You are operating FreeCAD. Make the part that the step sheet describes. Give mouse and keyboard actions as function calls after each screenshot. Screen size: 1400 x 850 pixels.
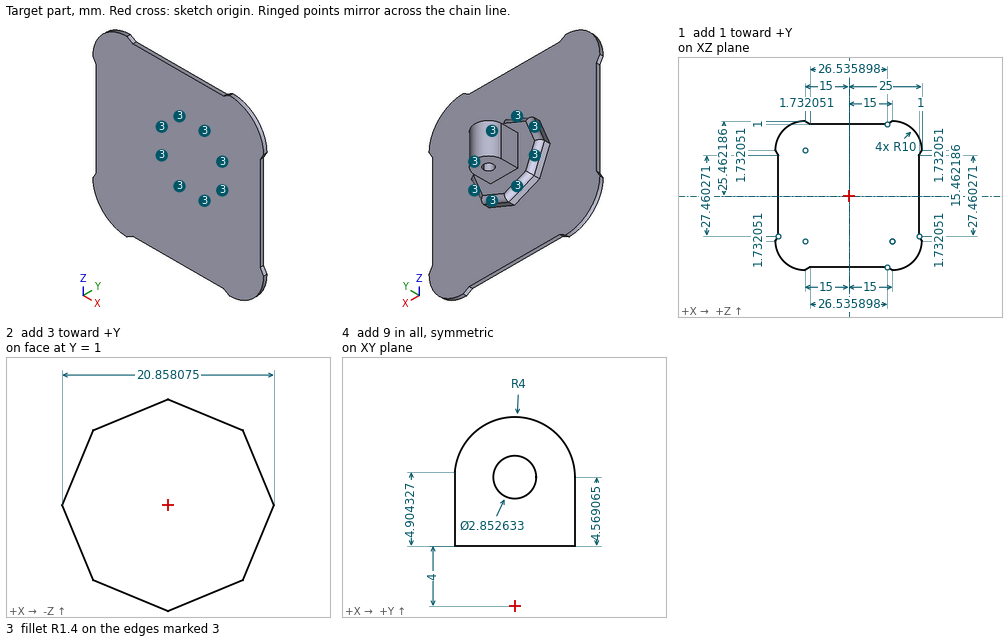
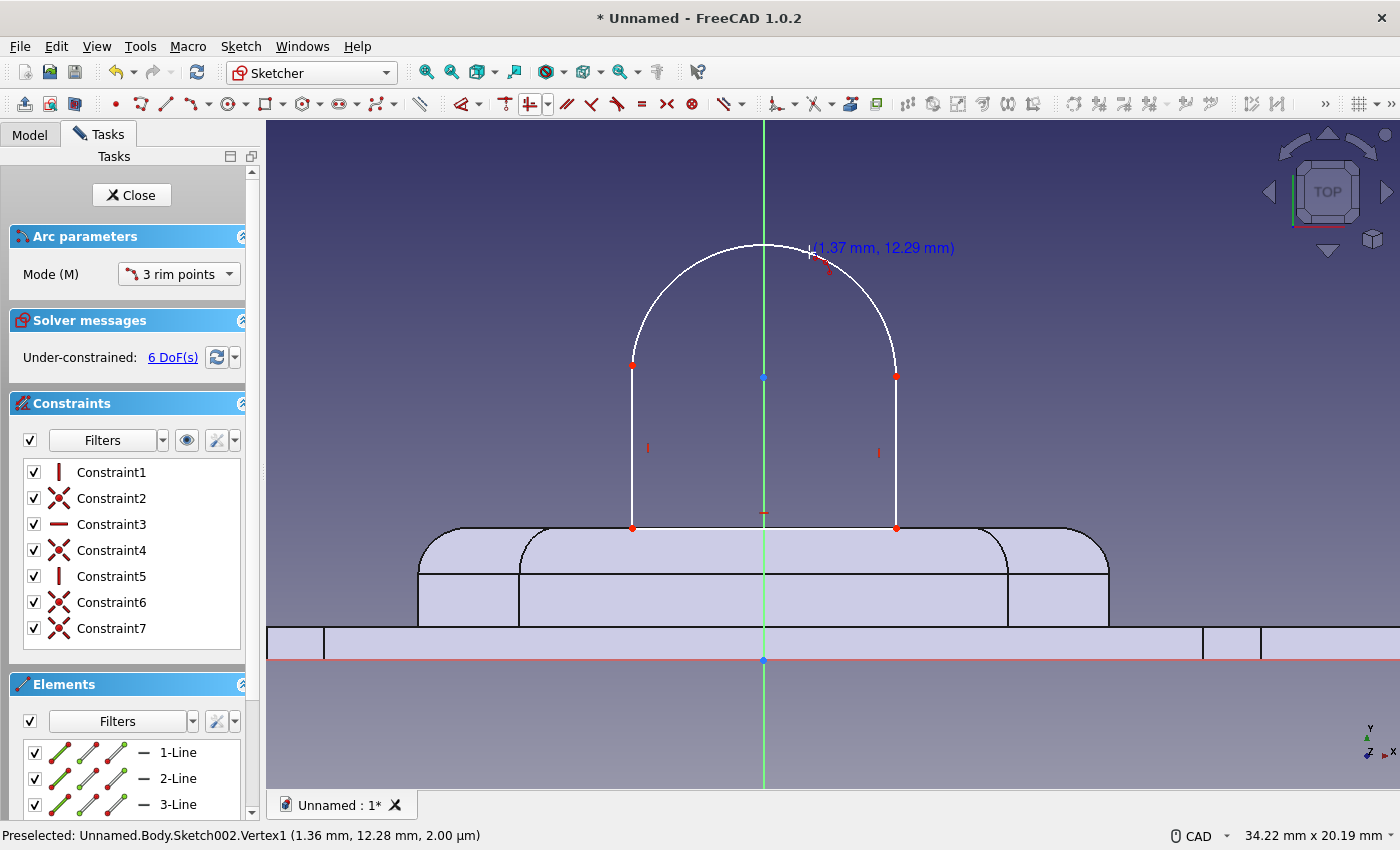
click(228, 104)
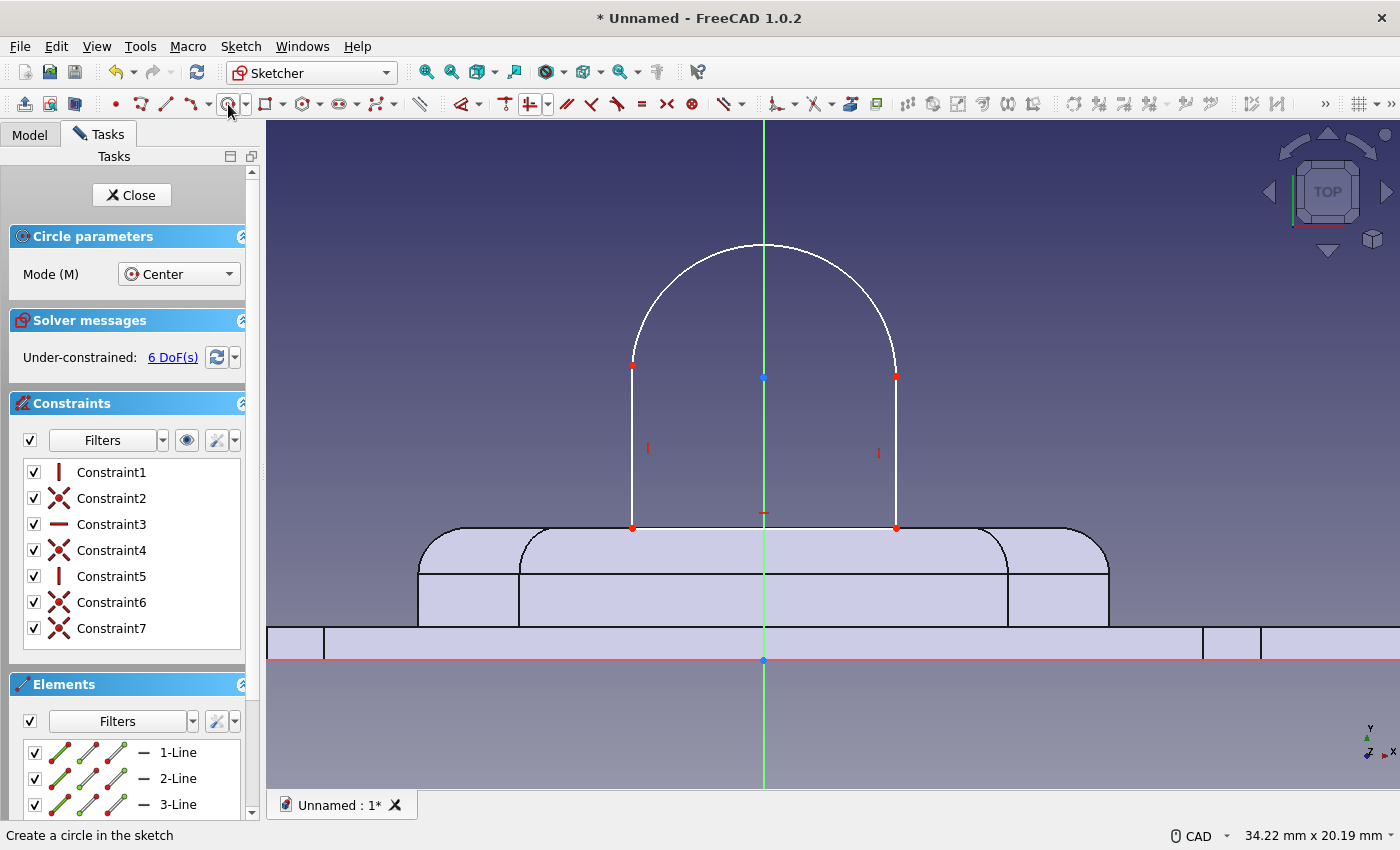
click(764, 376)
click(797, 343)
key(Escape)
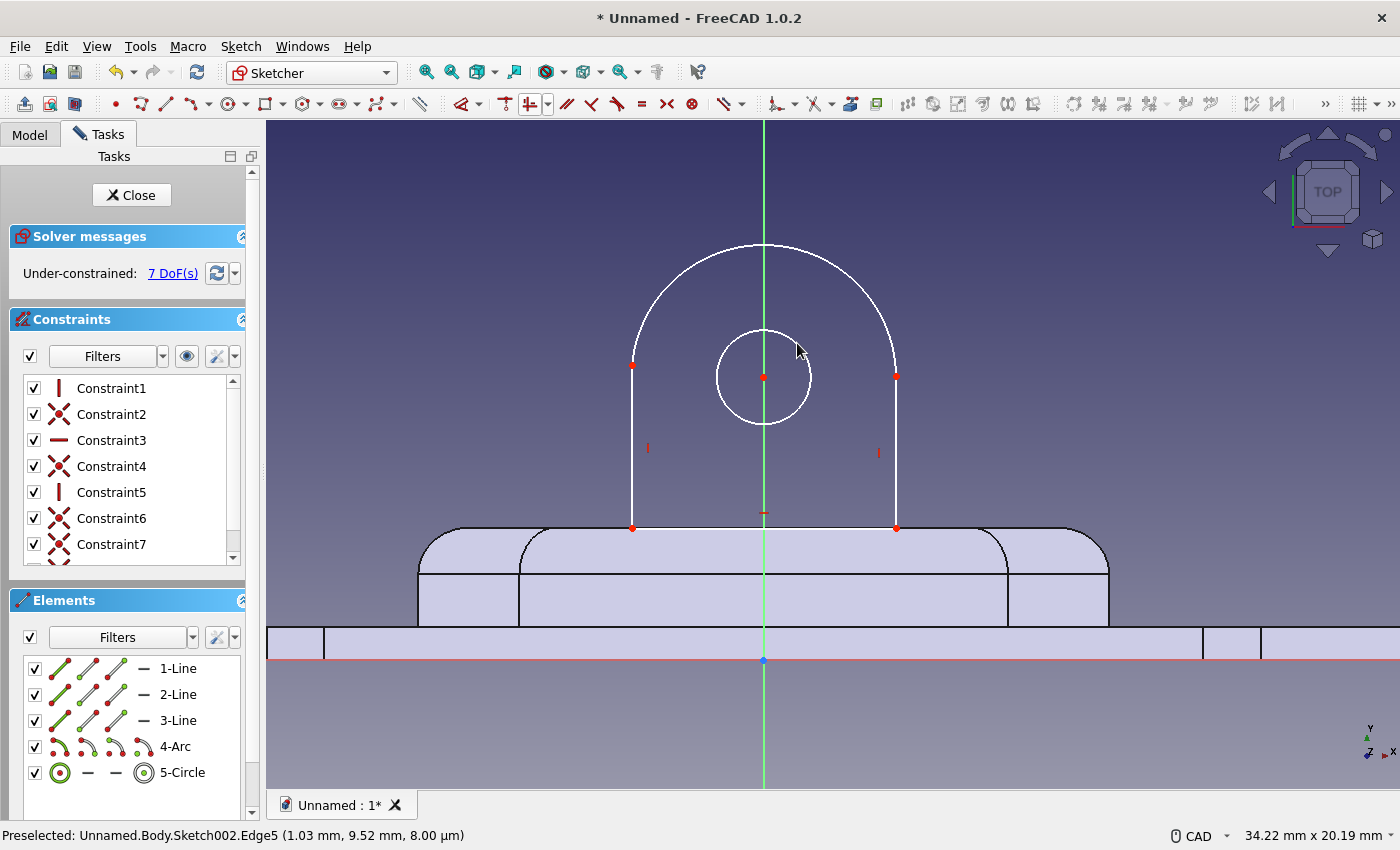
click(896, 483)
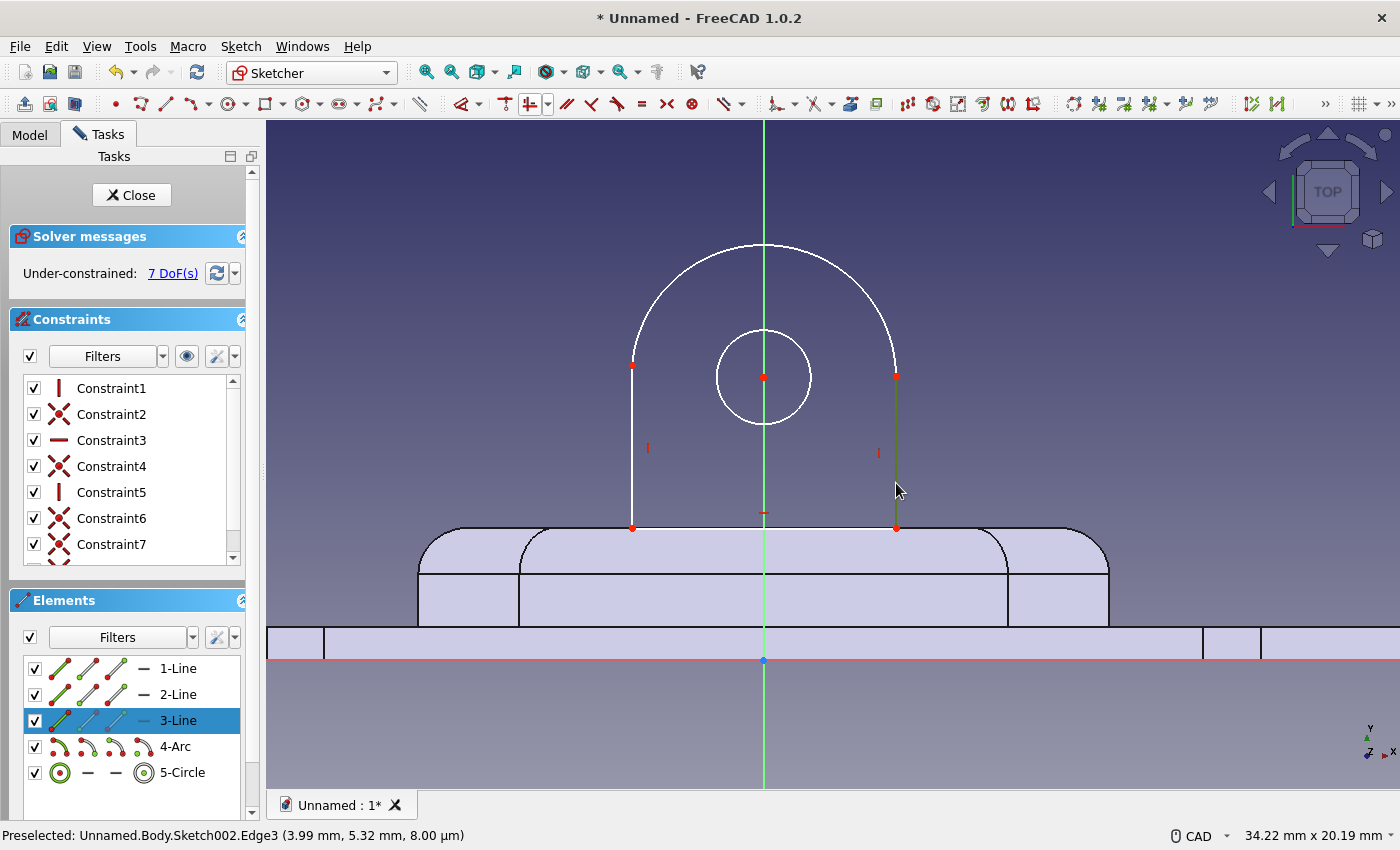
click(844, 272)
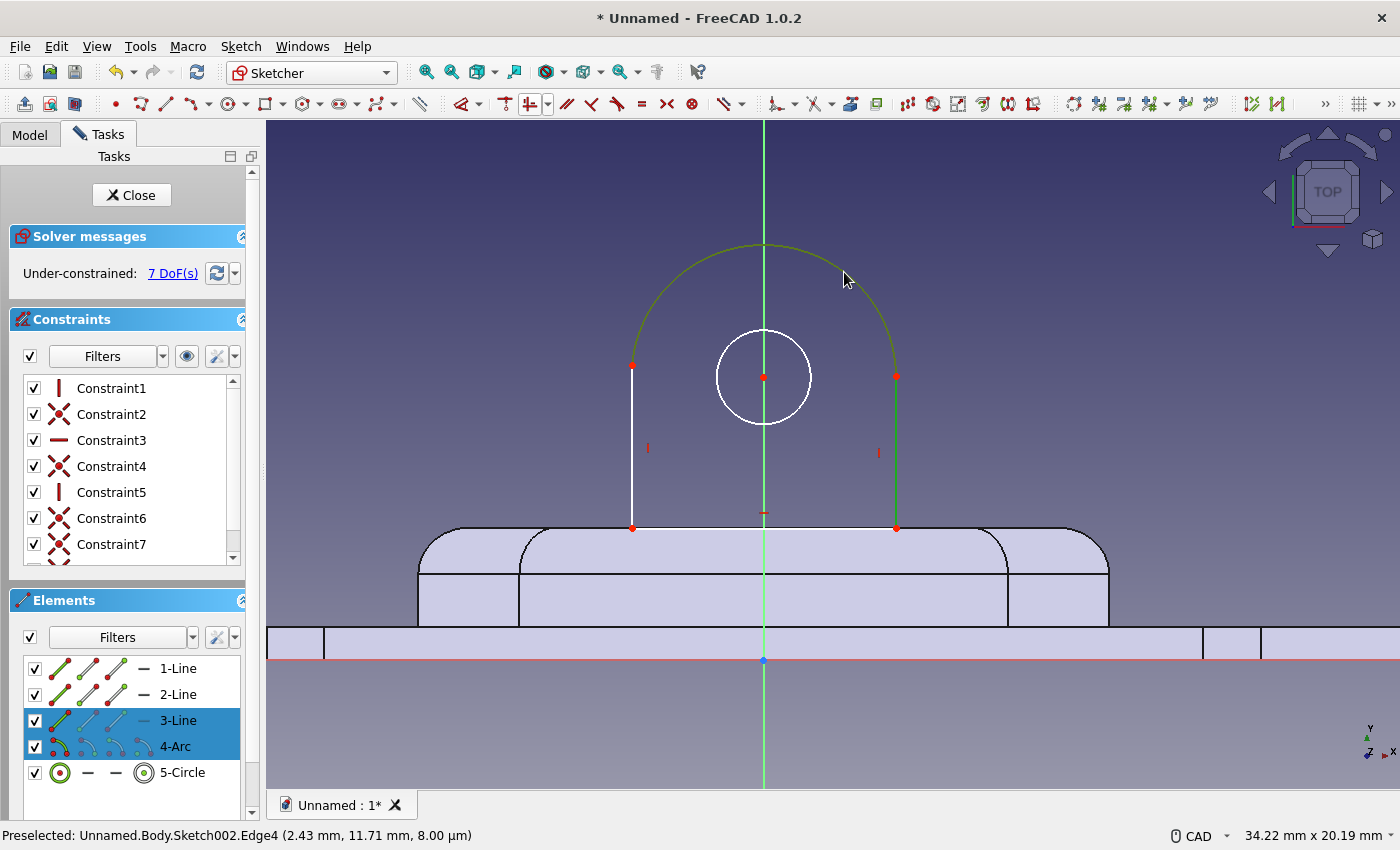
click(617, 104)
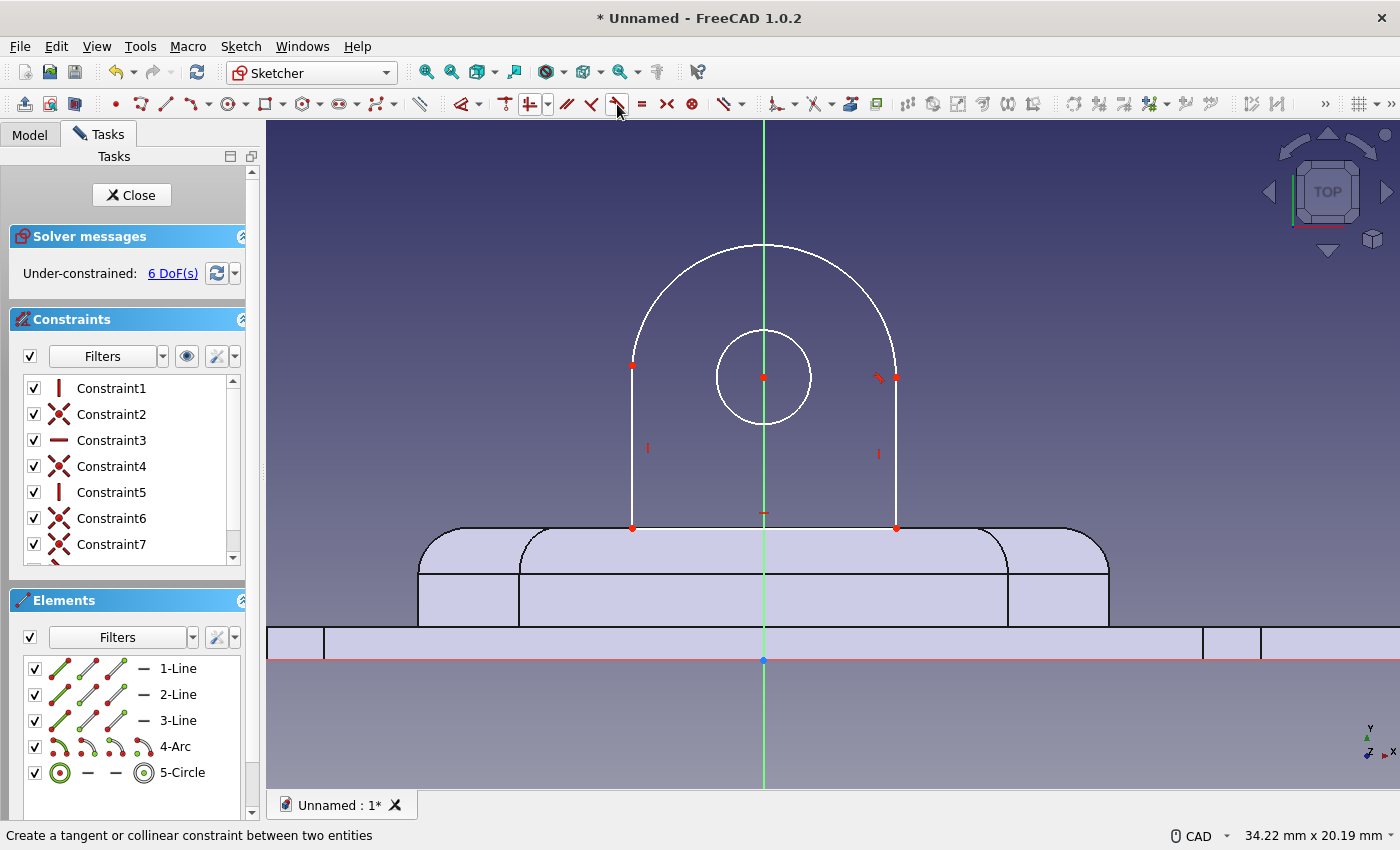
click(764, 377)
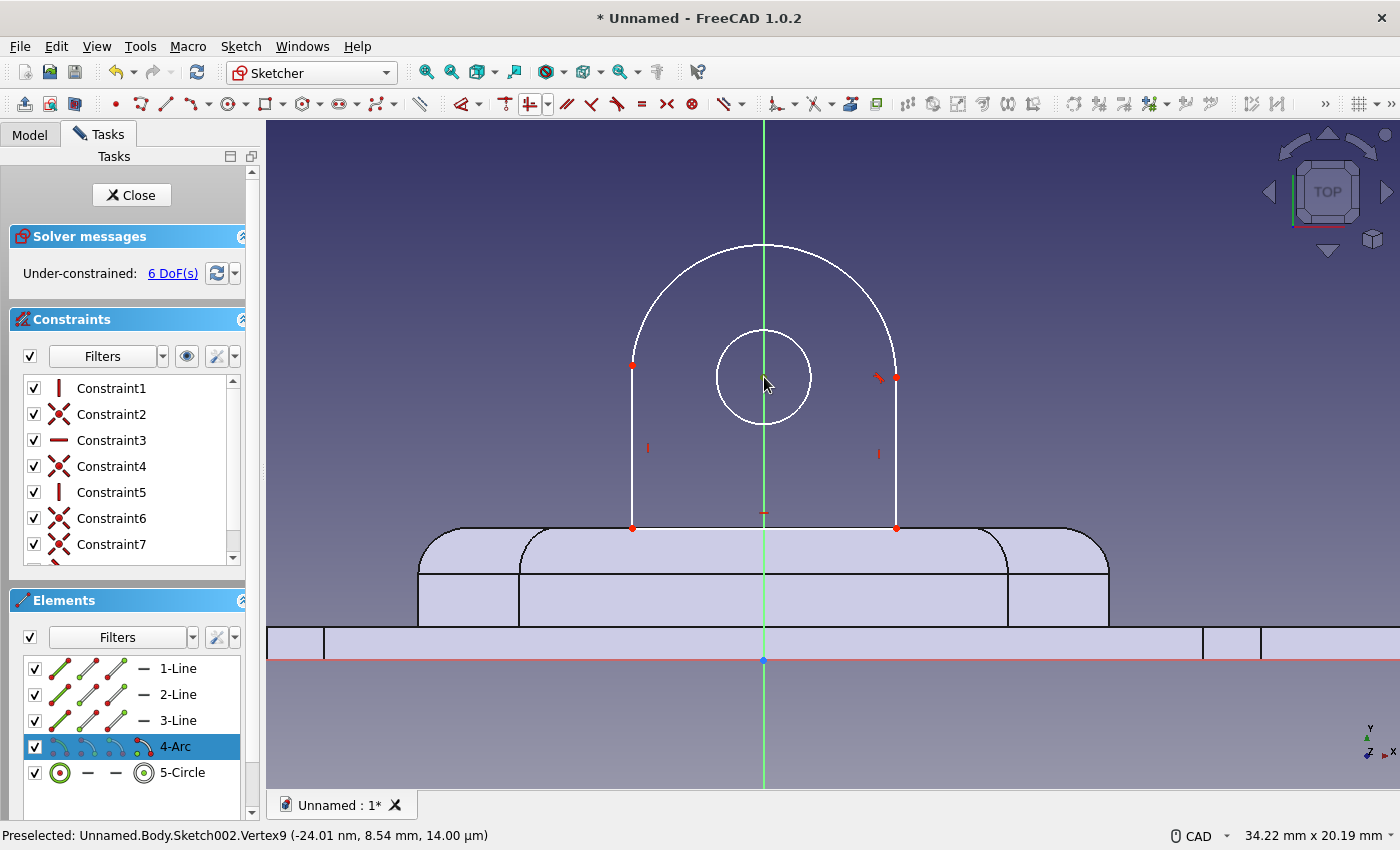
click(764, 717)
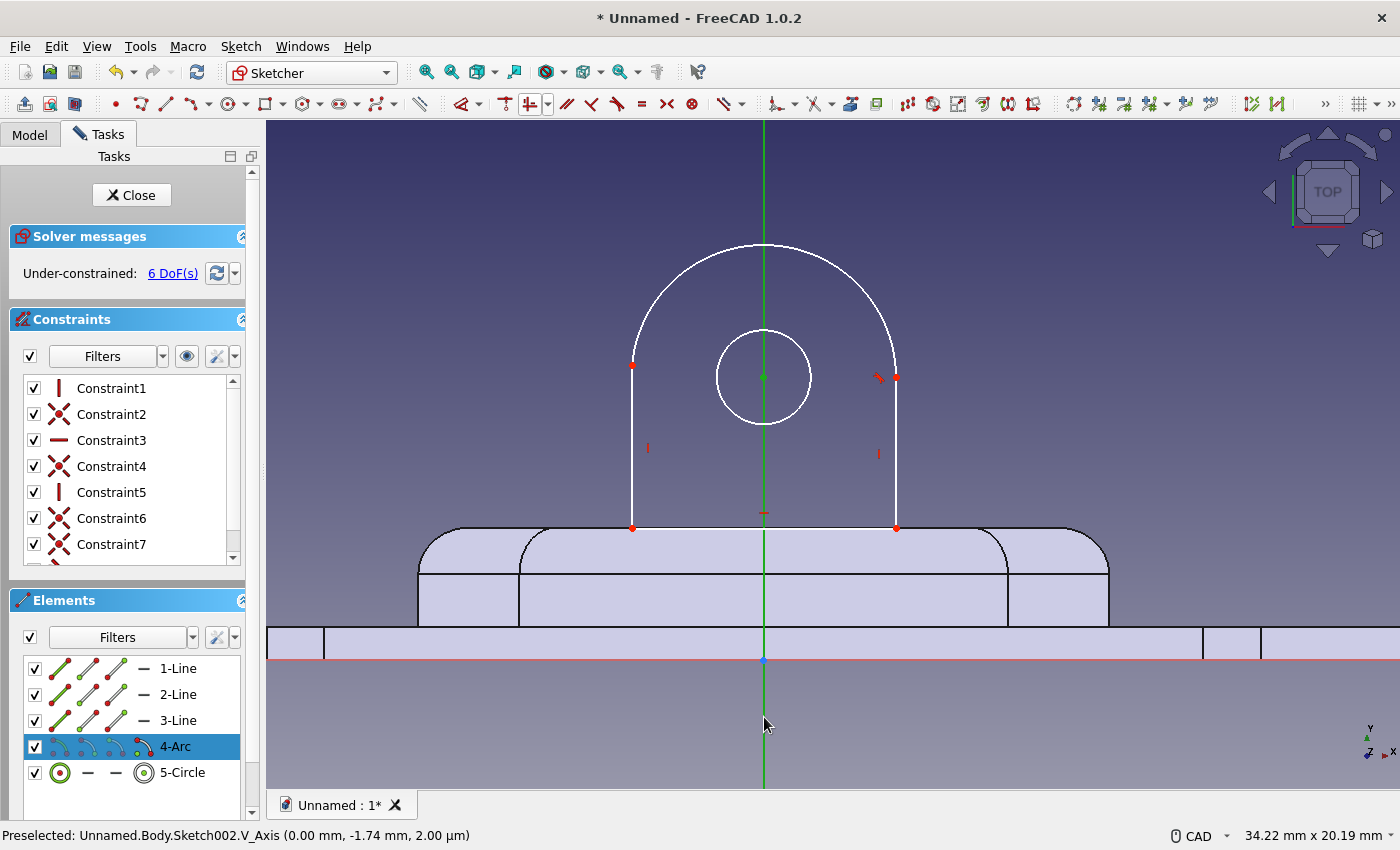
click(505, 104)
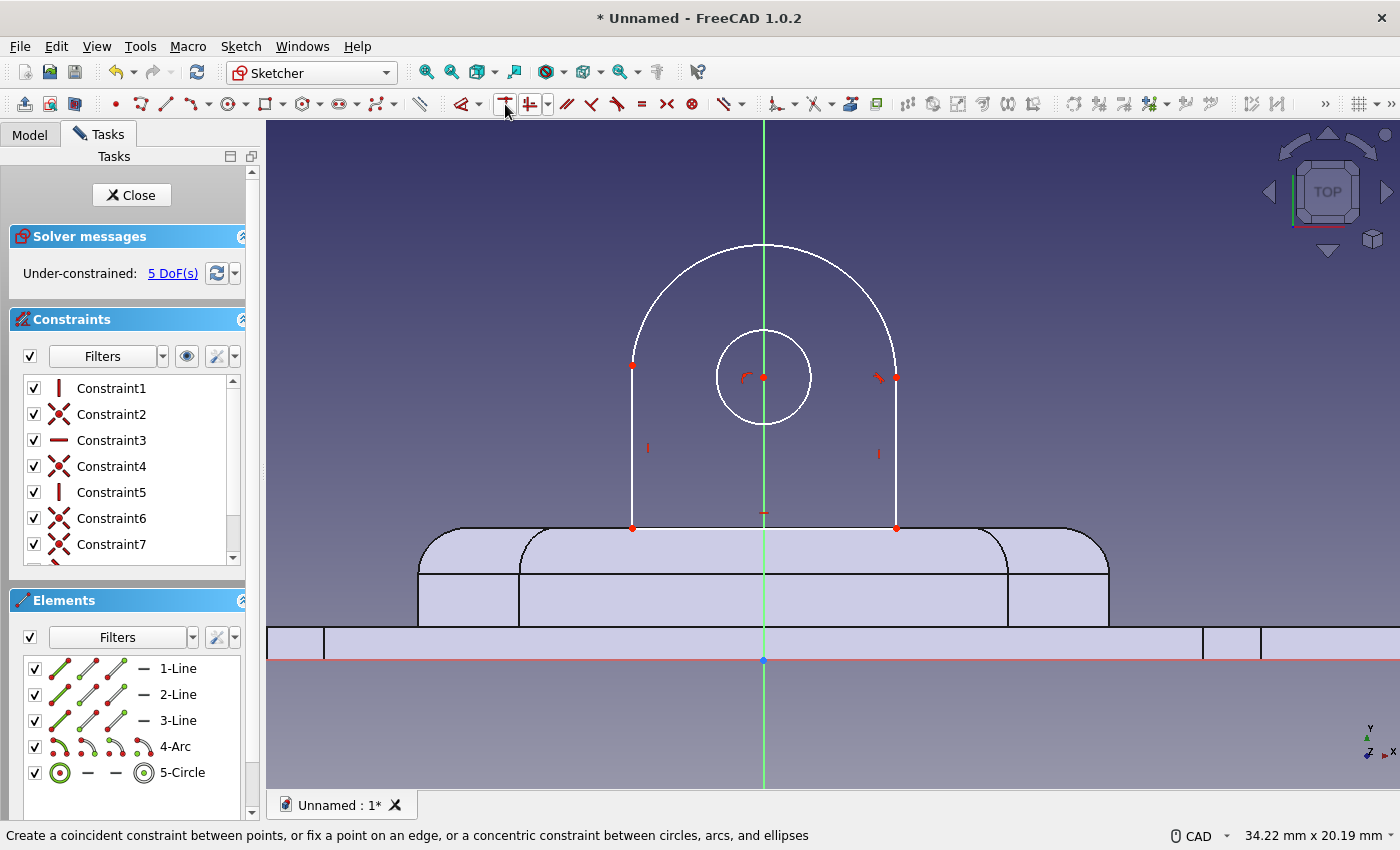
click(460, 104)